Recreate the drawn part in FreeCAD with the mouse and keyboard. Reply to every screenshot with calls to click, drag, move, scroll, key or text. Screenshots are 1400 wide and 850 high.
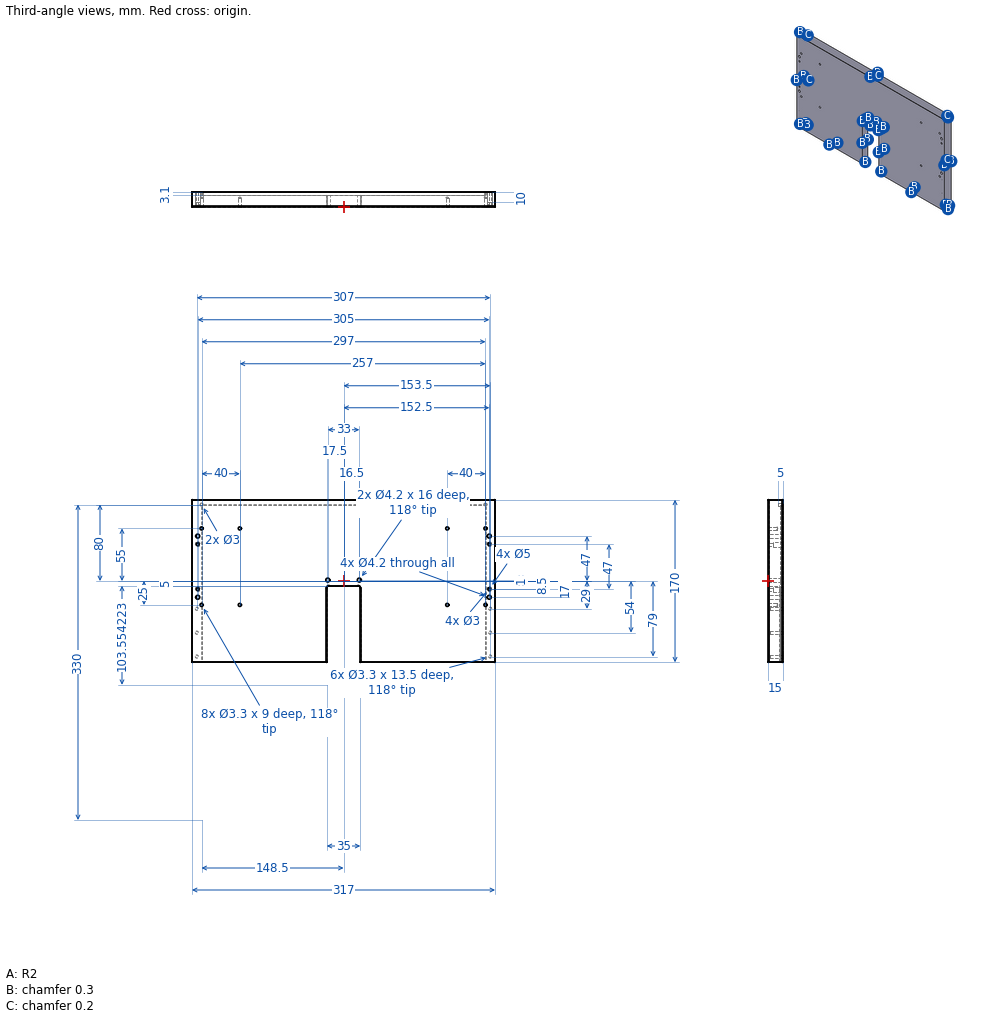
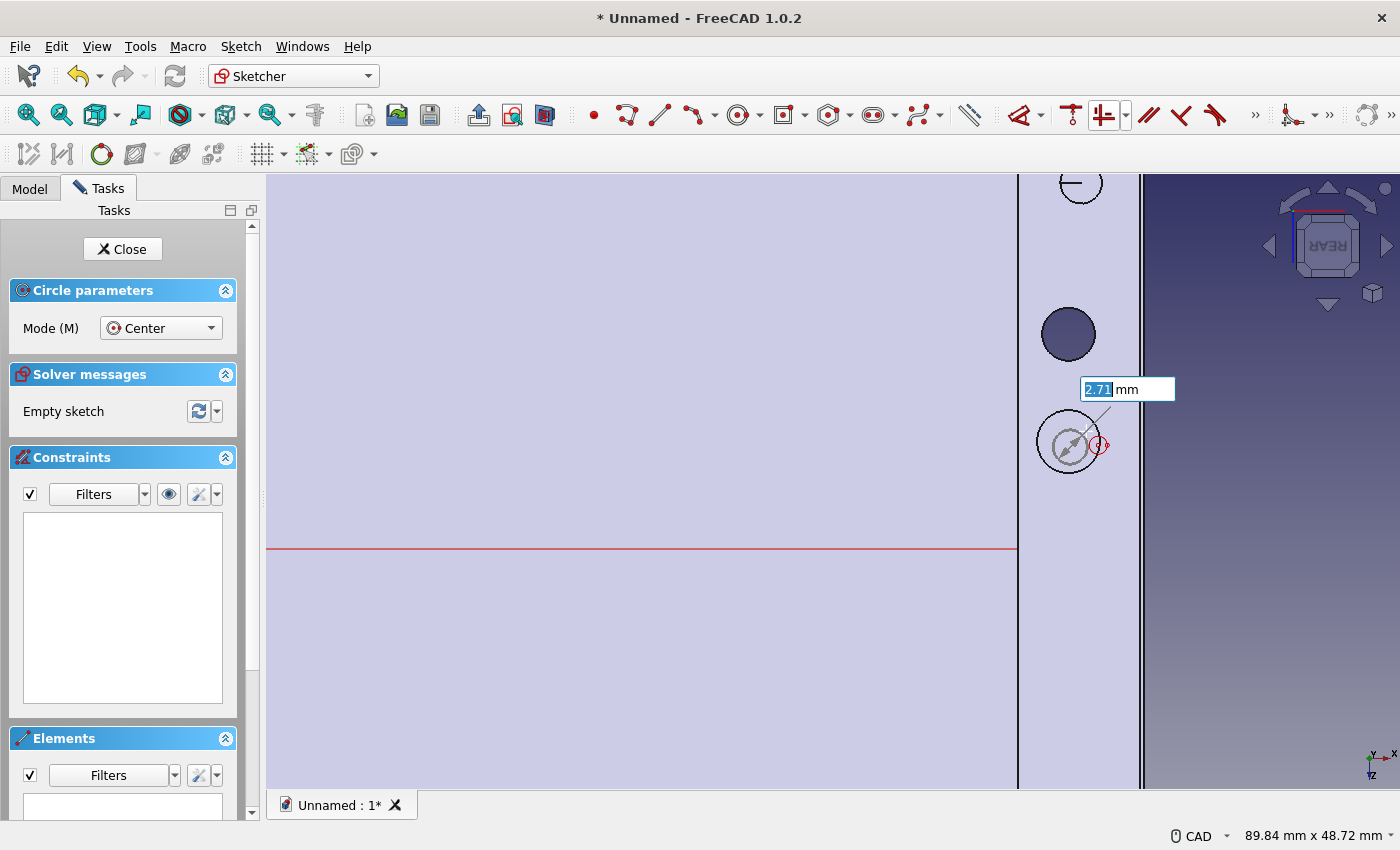
click(1082, 428)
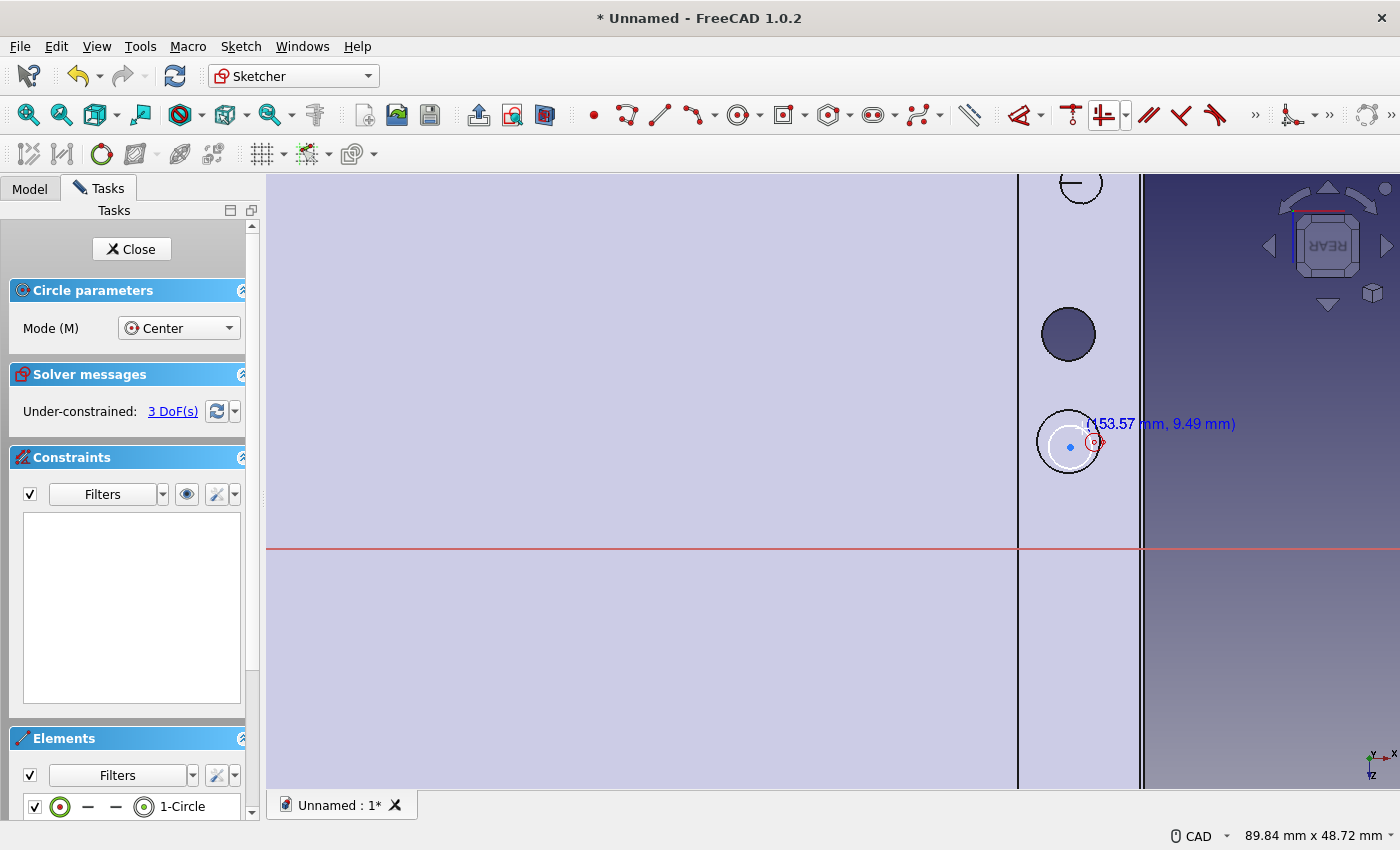
scroll(1085, 431, down, 9)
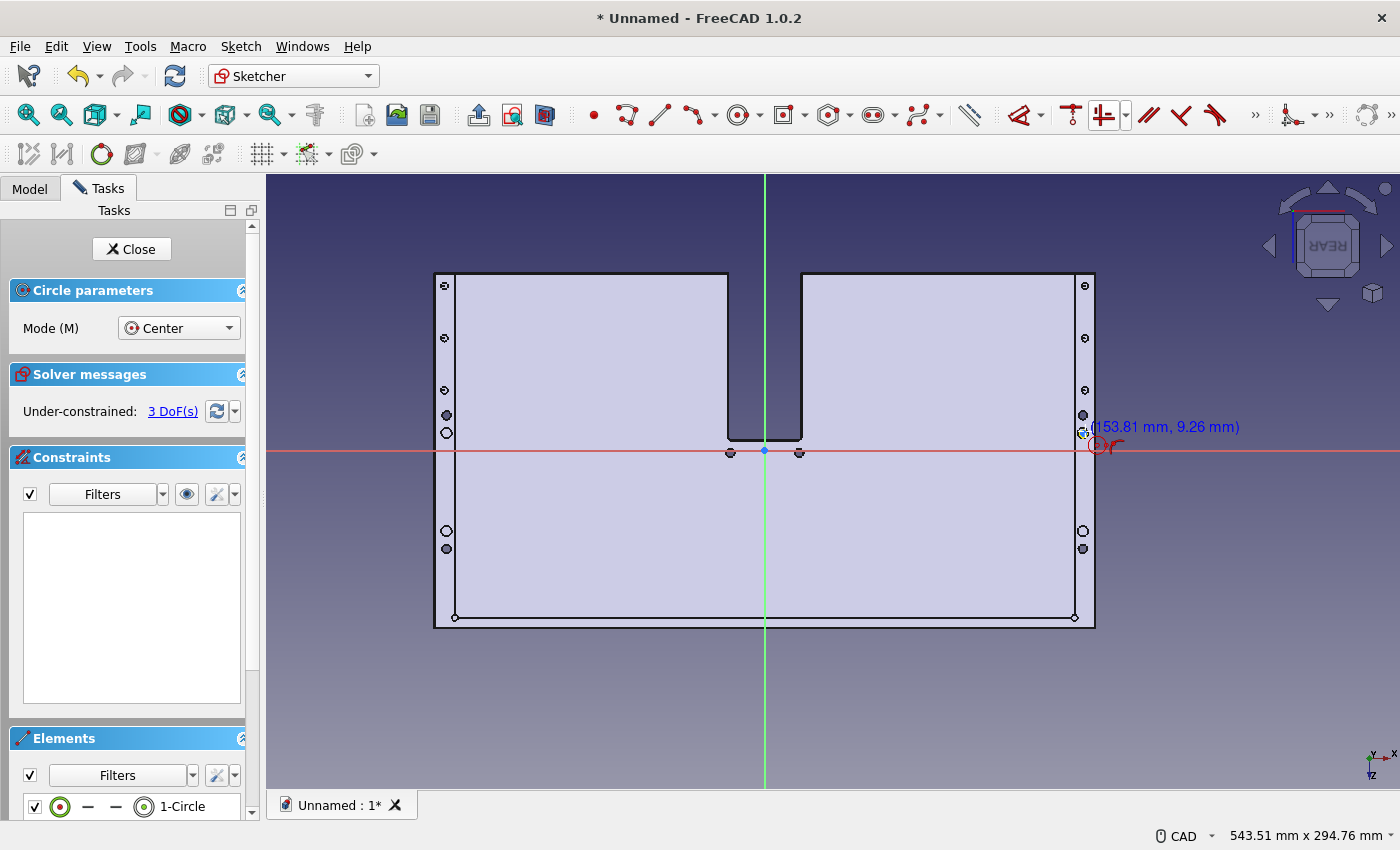
scroll(1083, 531, up, 10)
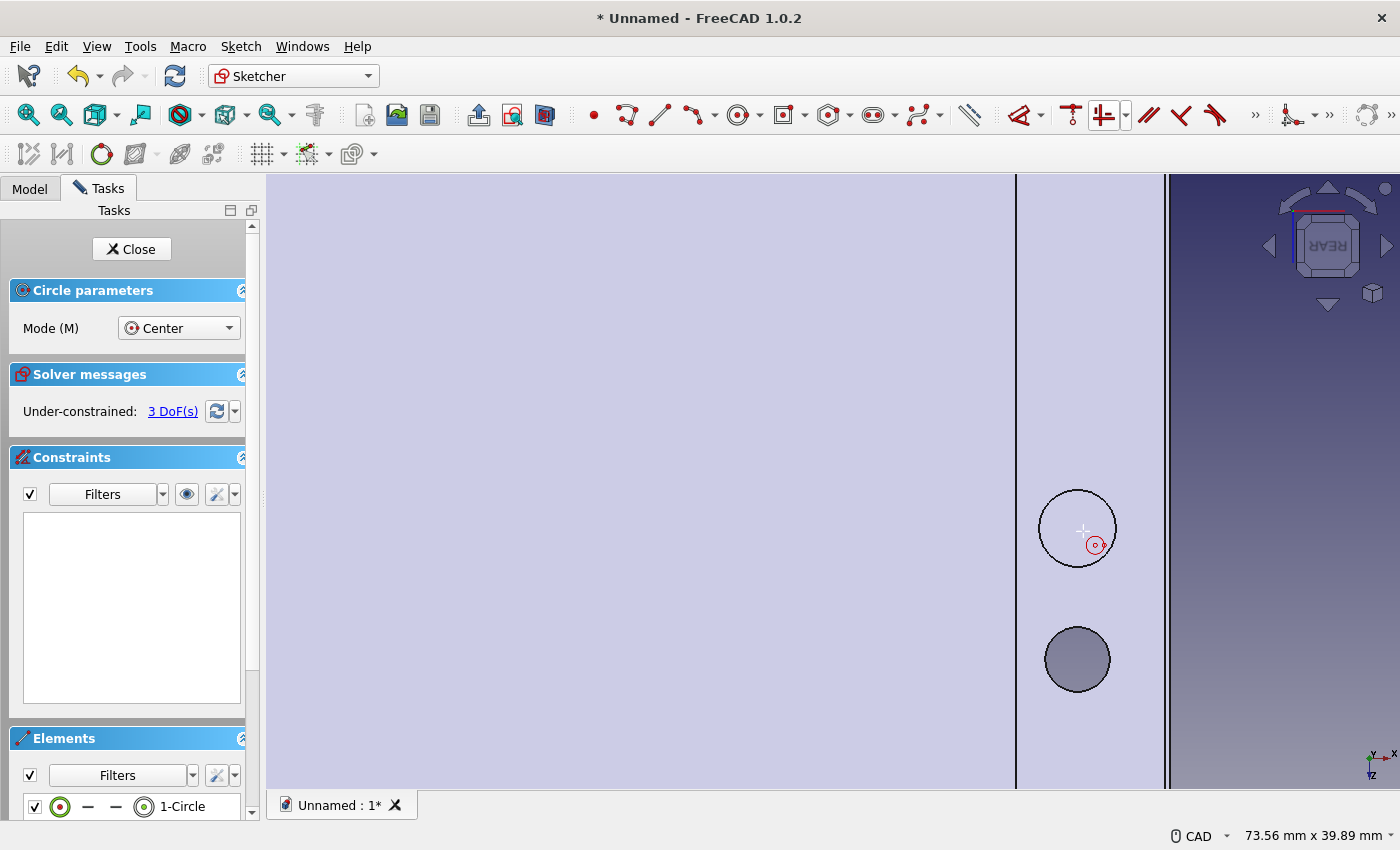
scroll(1083, 531, down, 10)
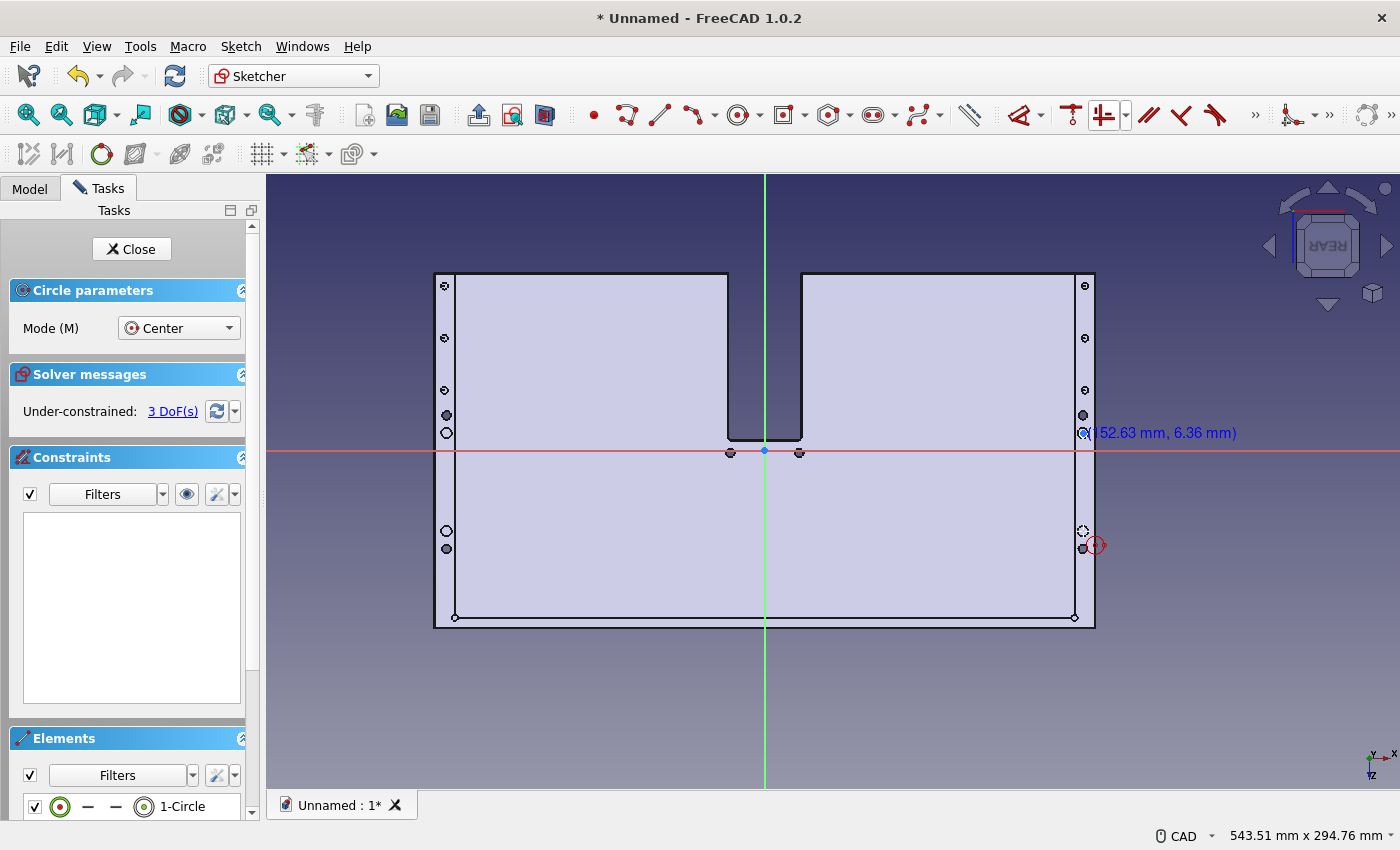
click(1083, 531)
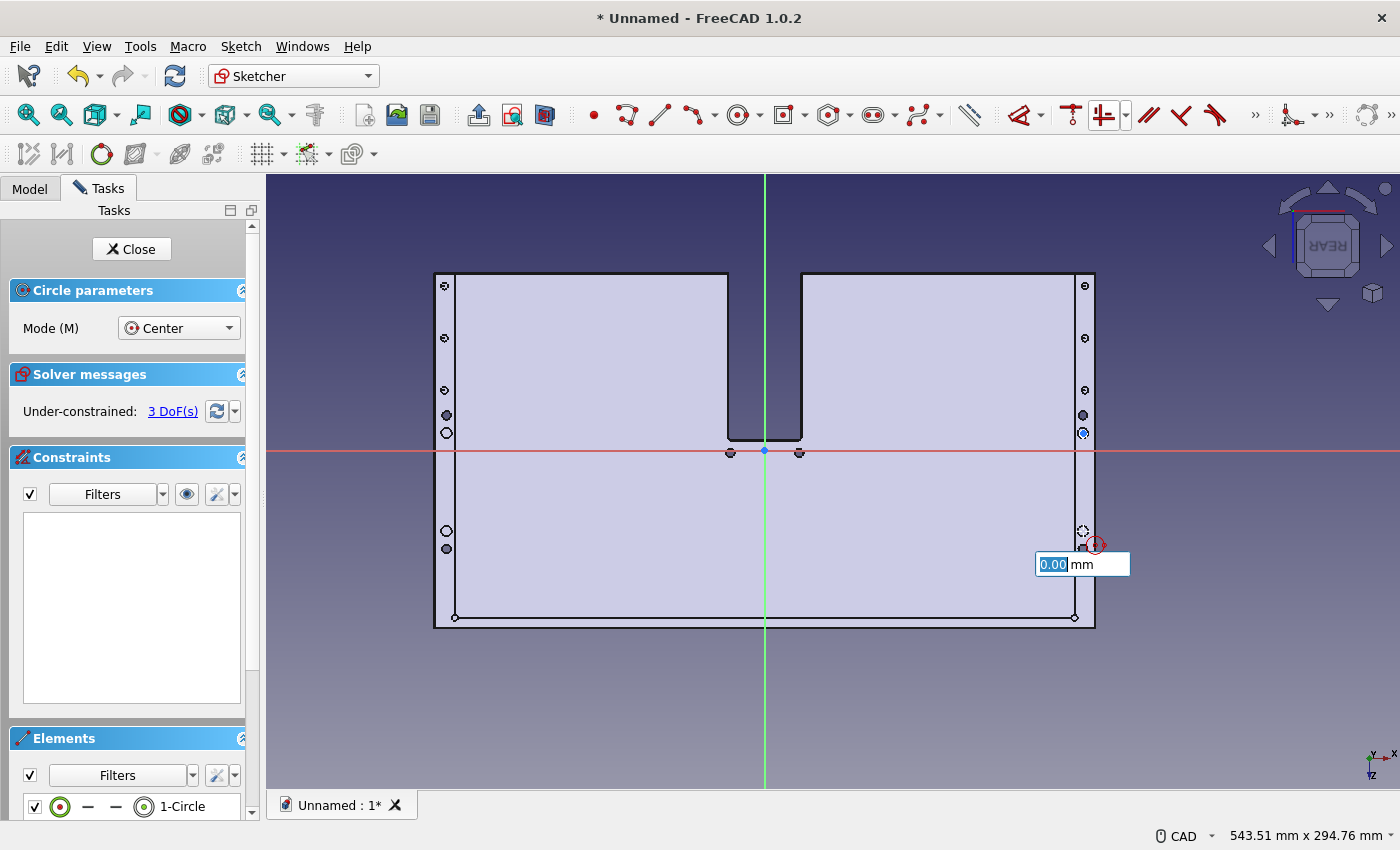
scroll(1085, 529, up, 9)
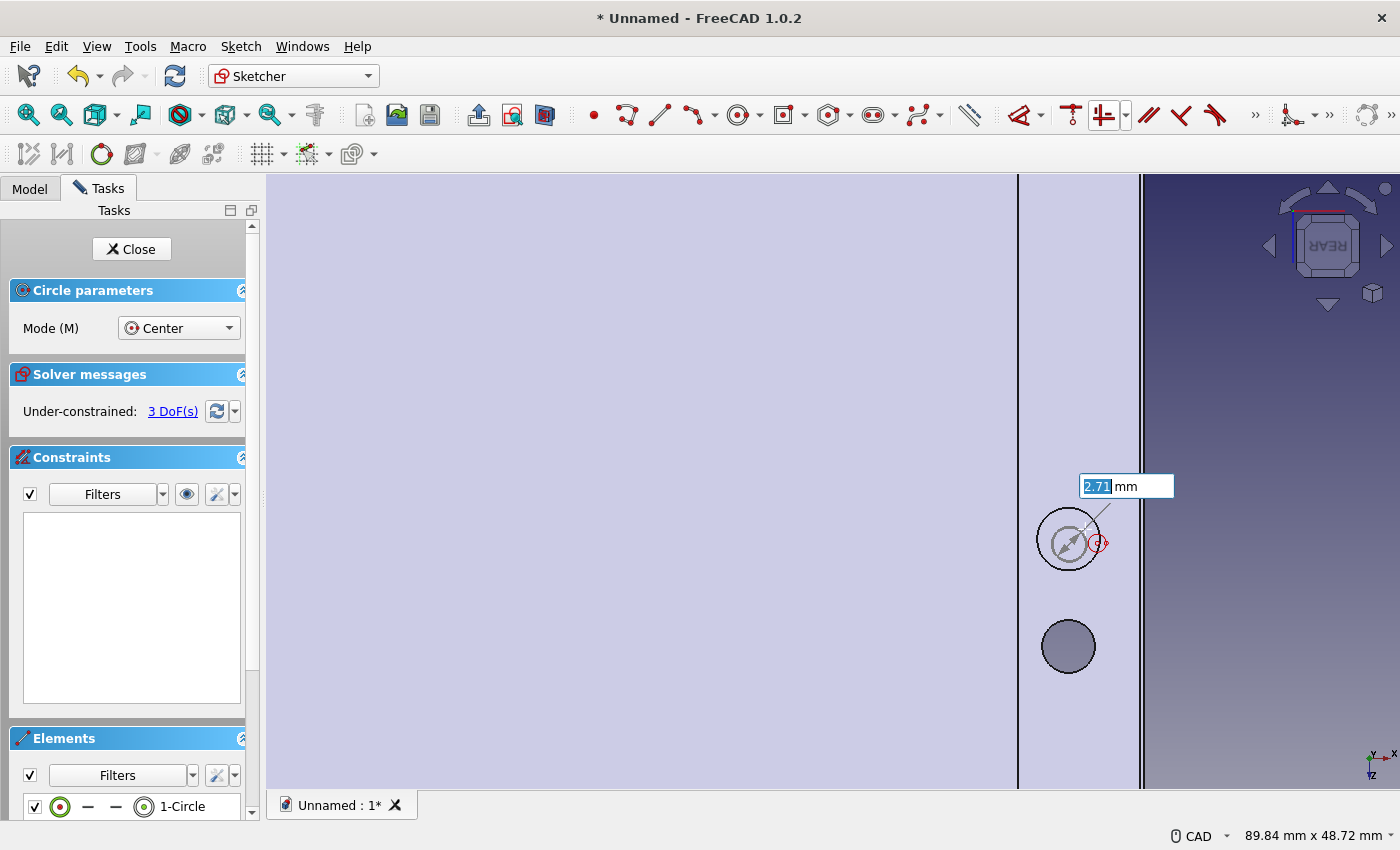
click(1082, 526)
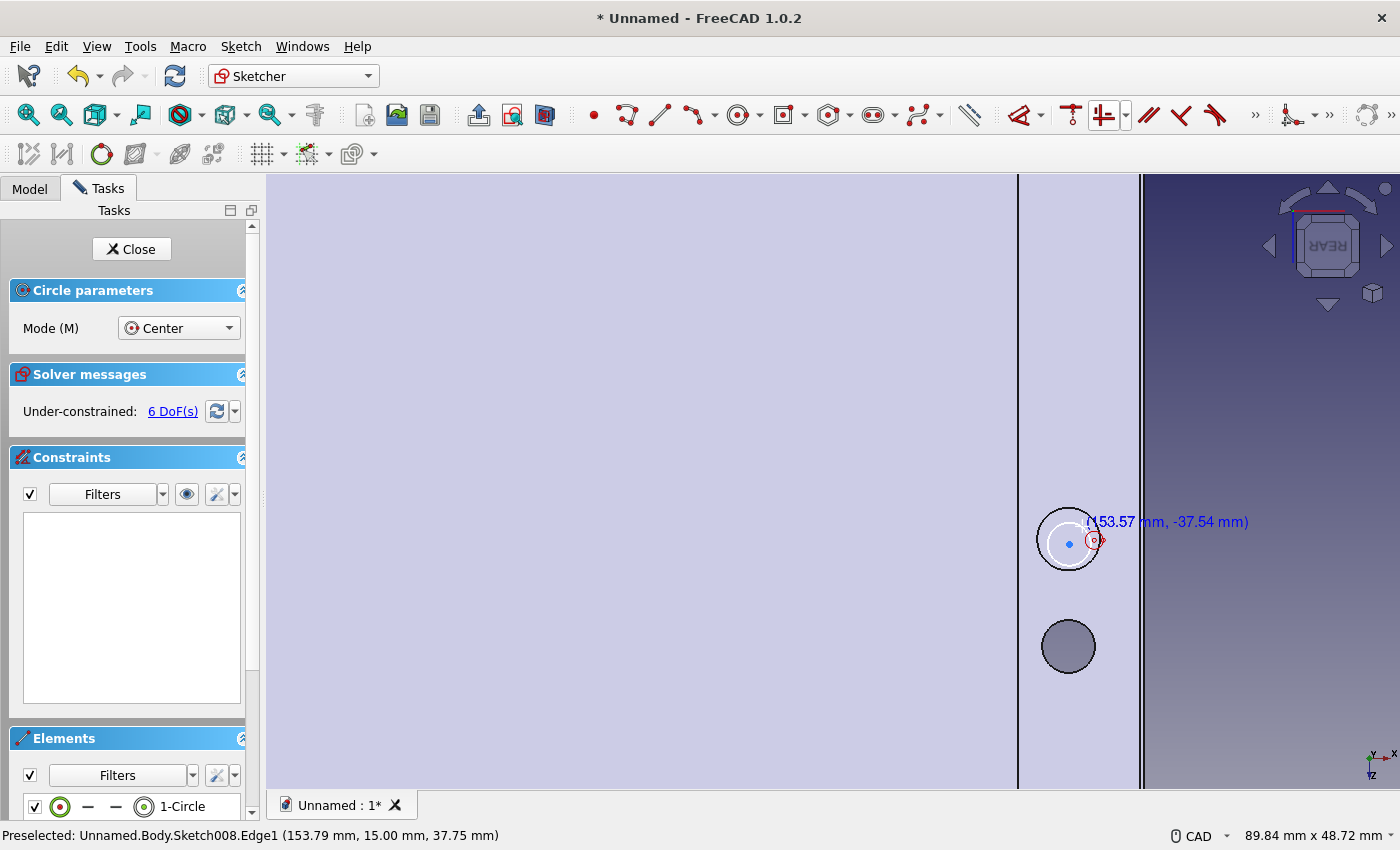
scroll(1085, 529, down, 9)